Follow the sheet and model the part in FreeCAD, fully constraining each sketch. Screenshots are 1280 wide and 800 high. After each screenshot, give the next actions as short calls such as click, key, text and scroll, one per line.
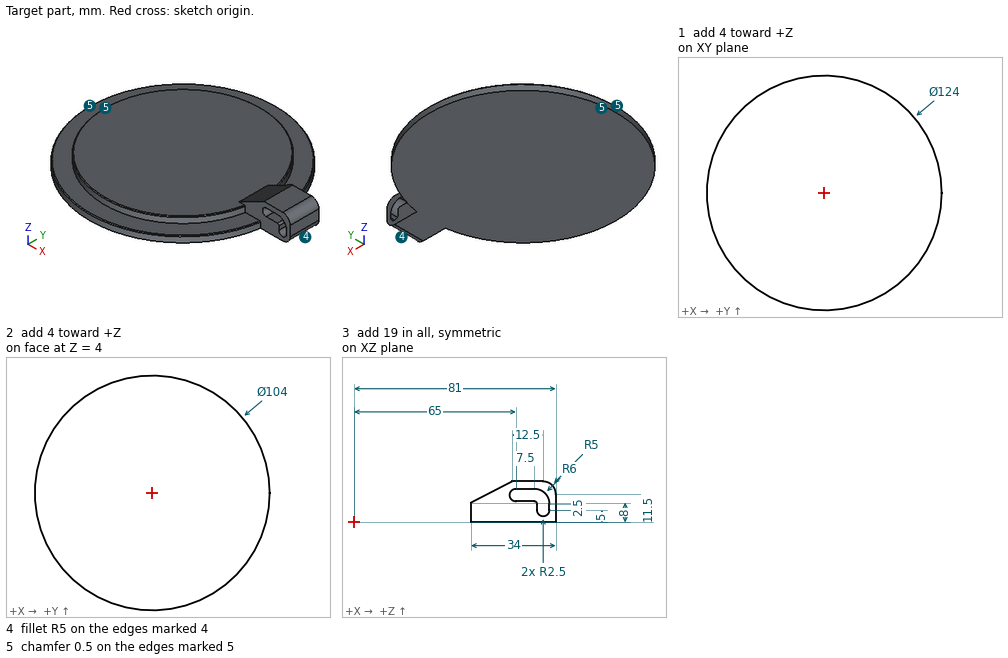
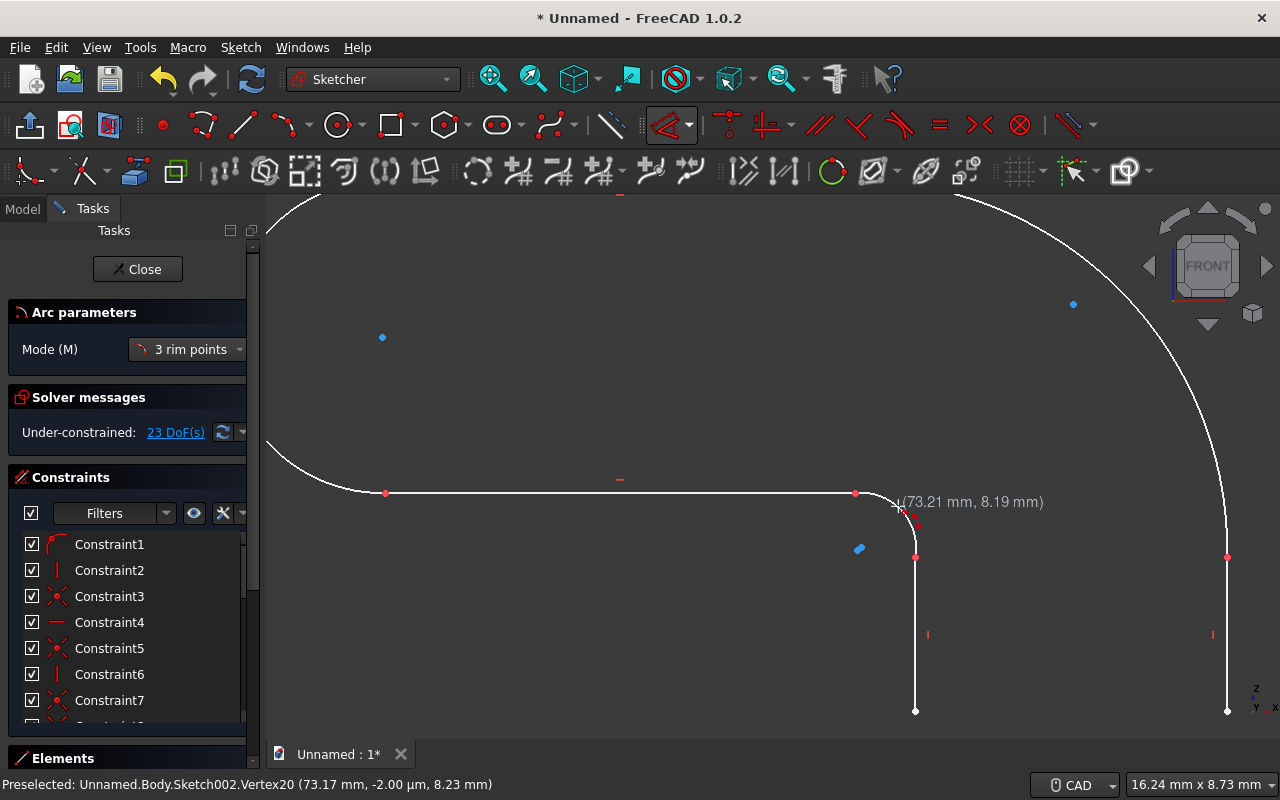
scroll(935, 462, down, 11)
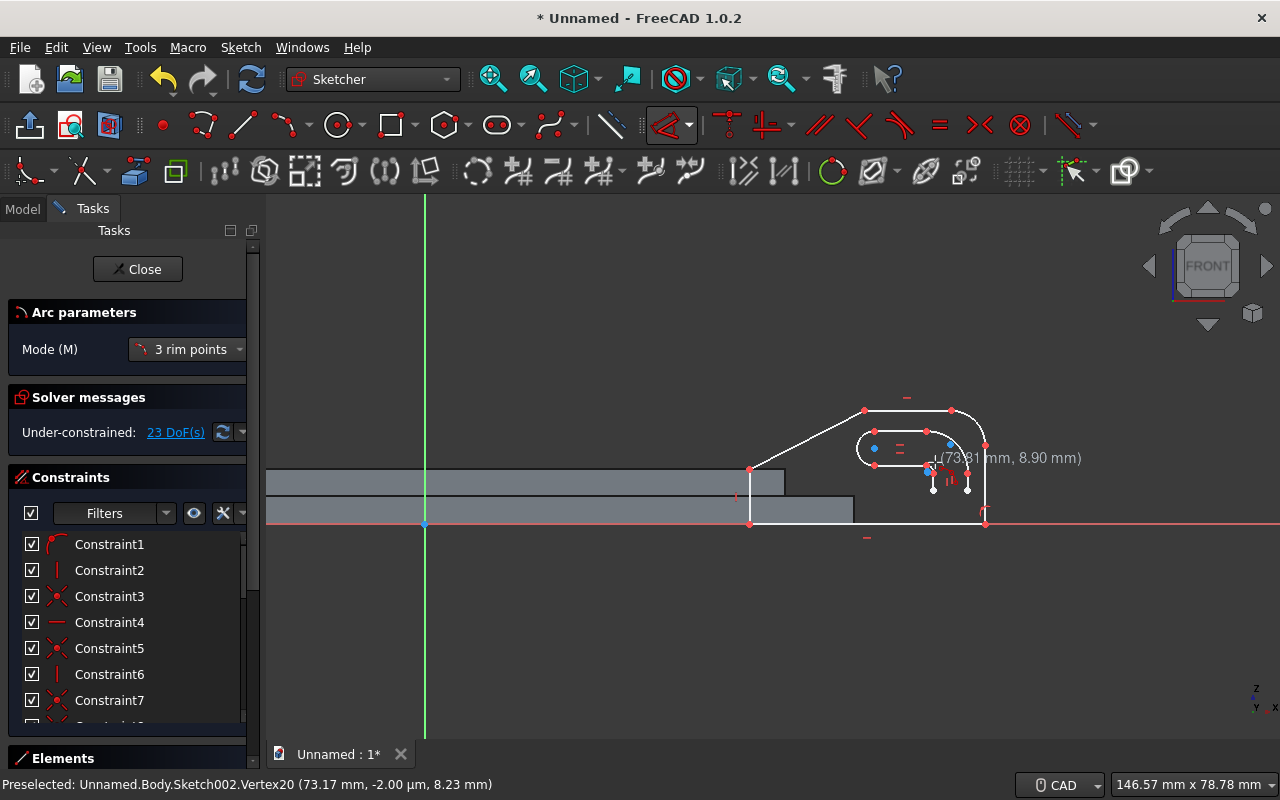
scroll(933, 490, up, 4)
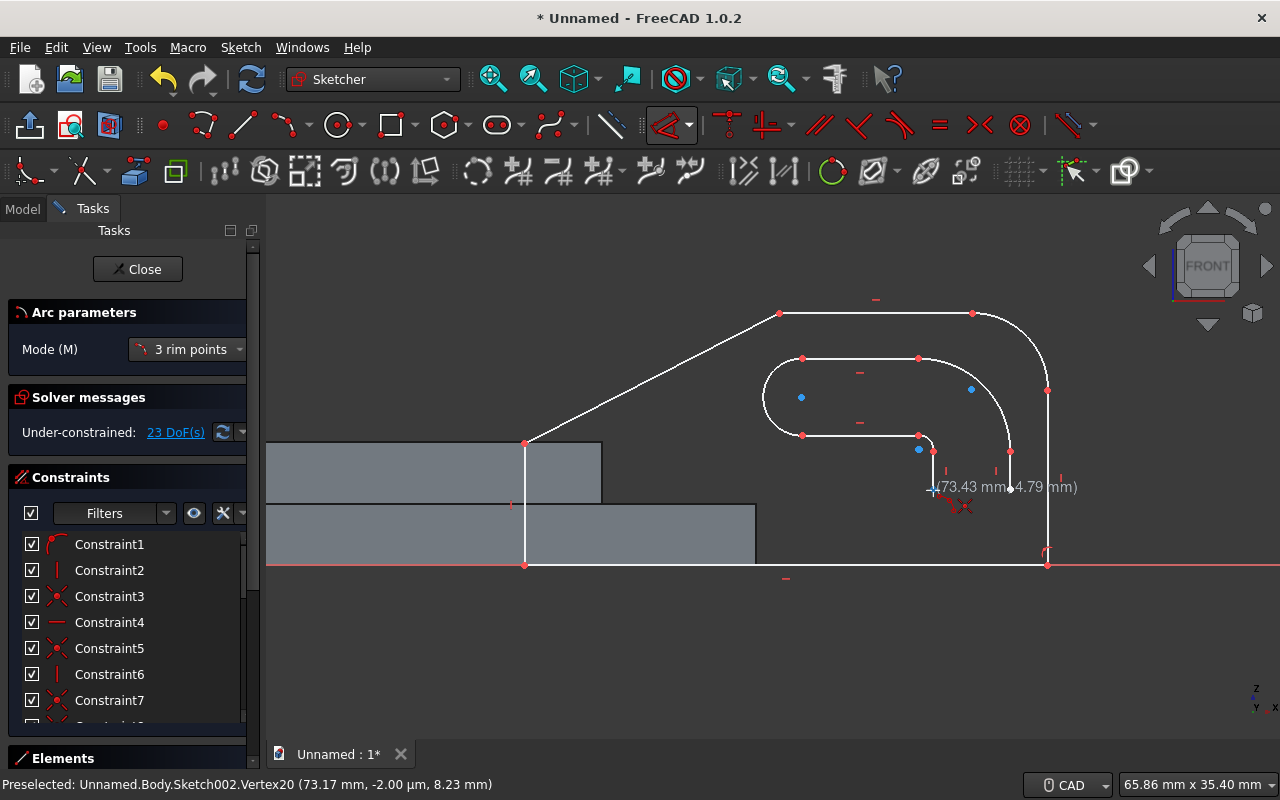
click(933, 489)
click(1010, 489)
click(972, 527)
key(Escape)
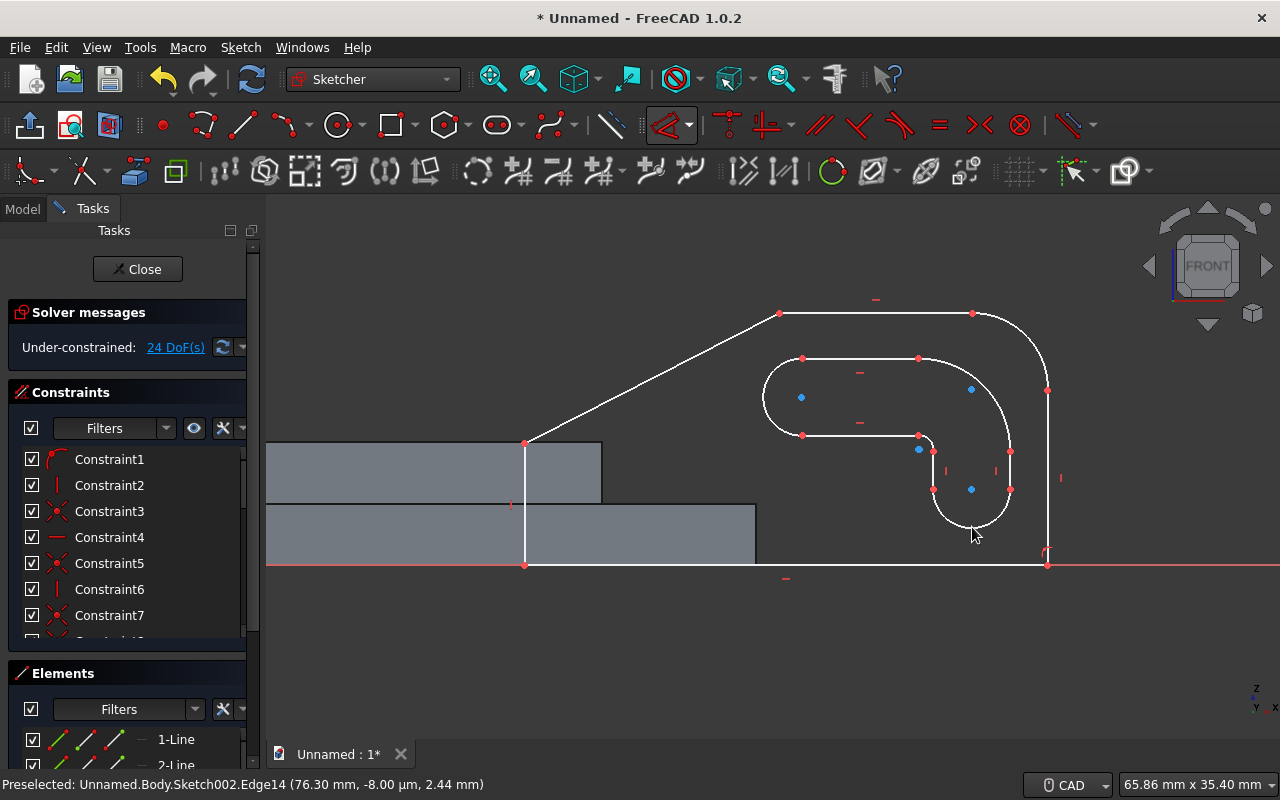
click(1048, 443)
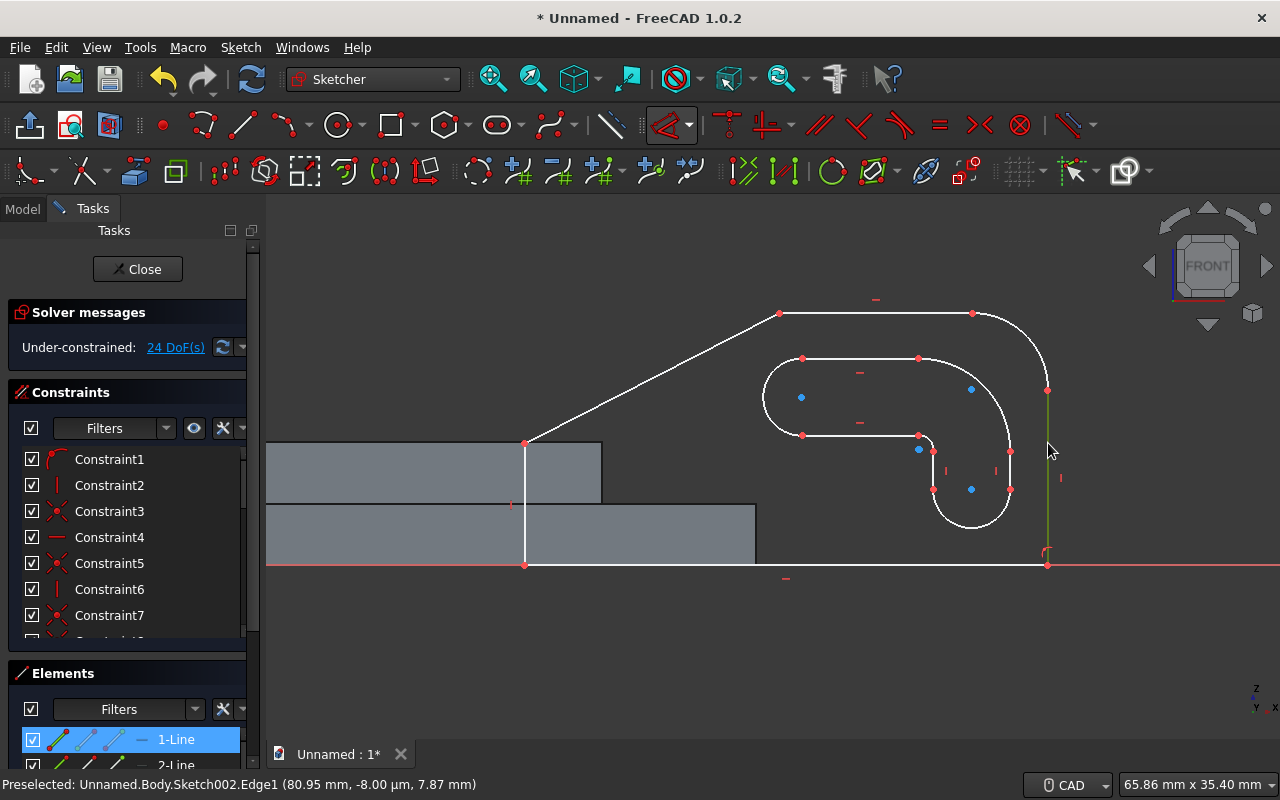
click(1040, 356)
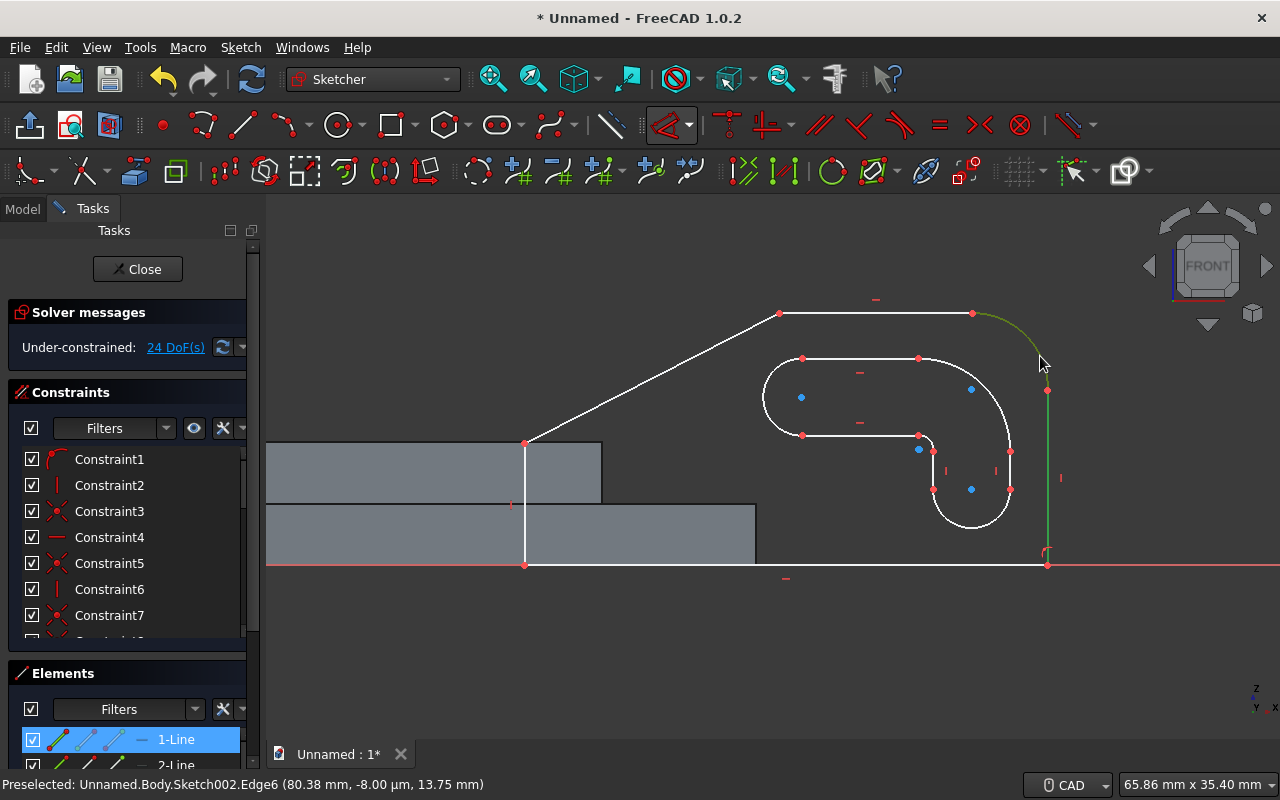
click(900, 126)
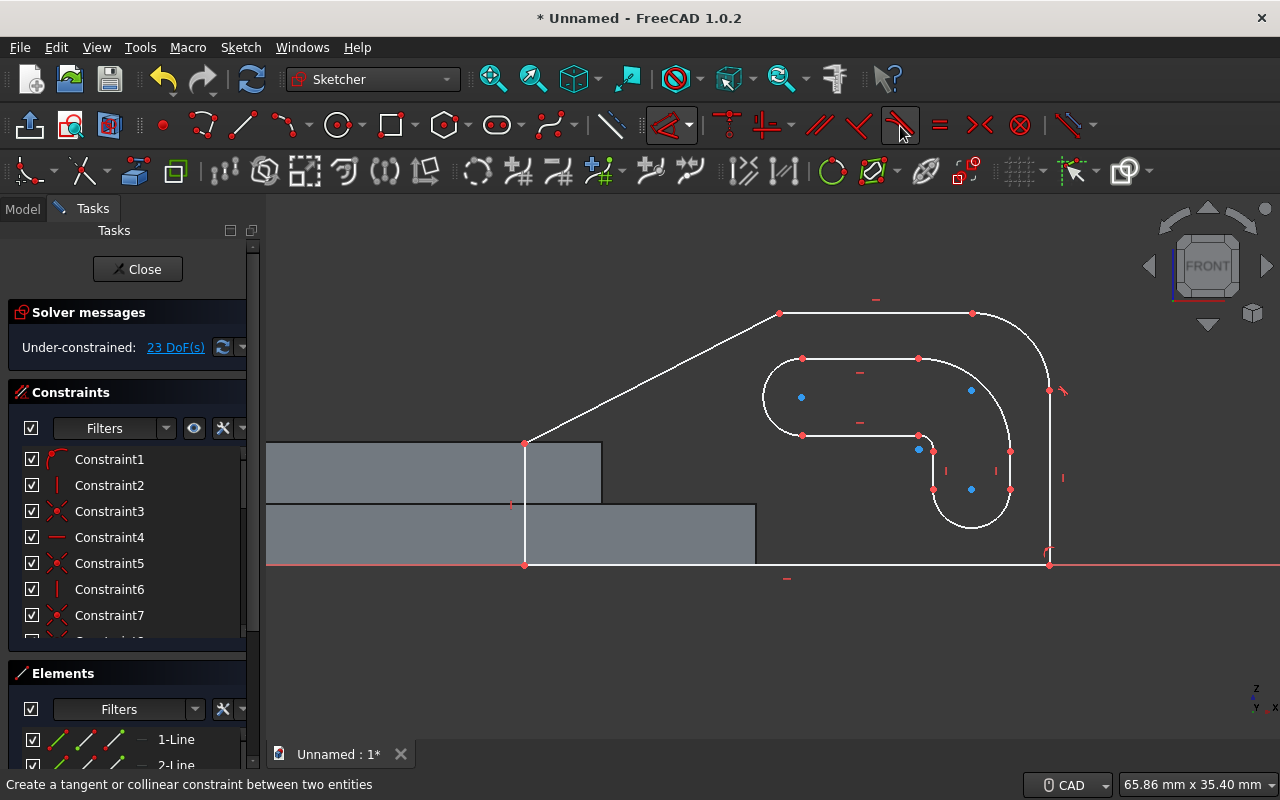
click(838, 313)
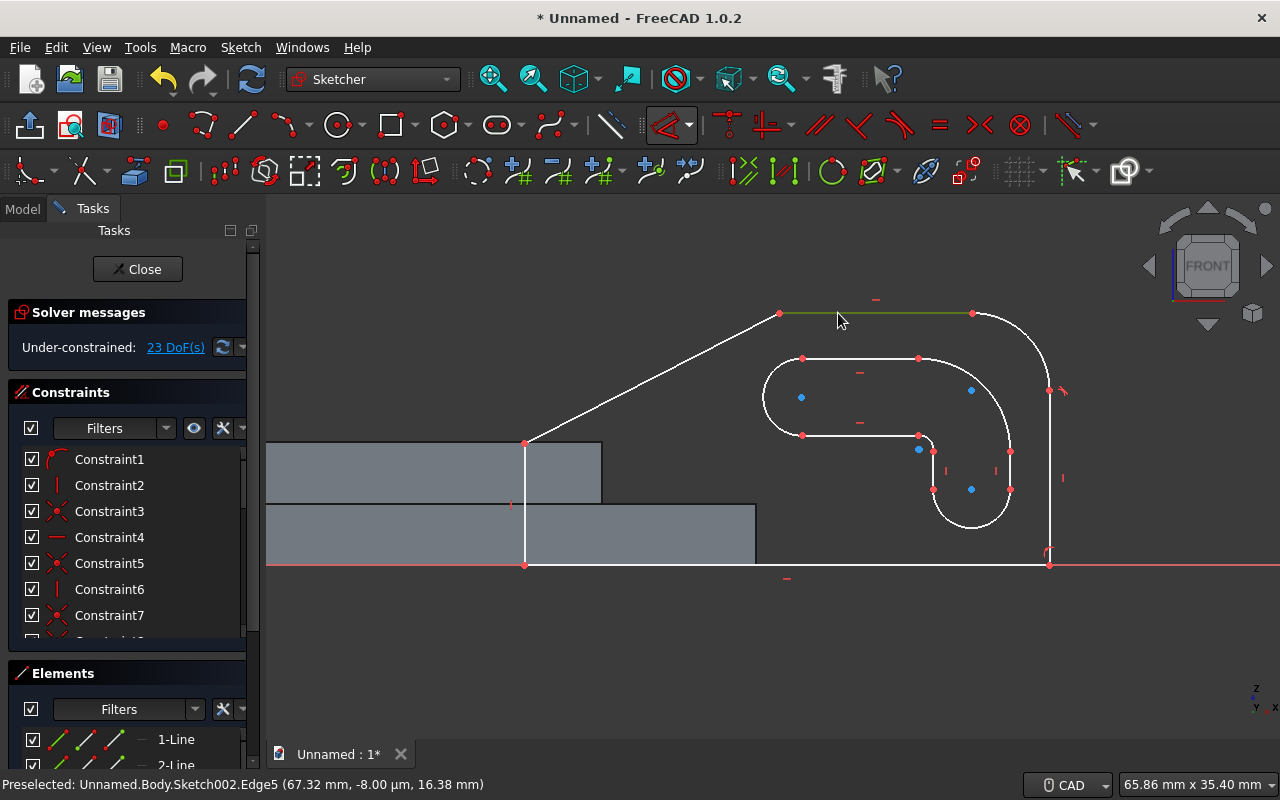
click(1041, 356)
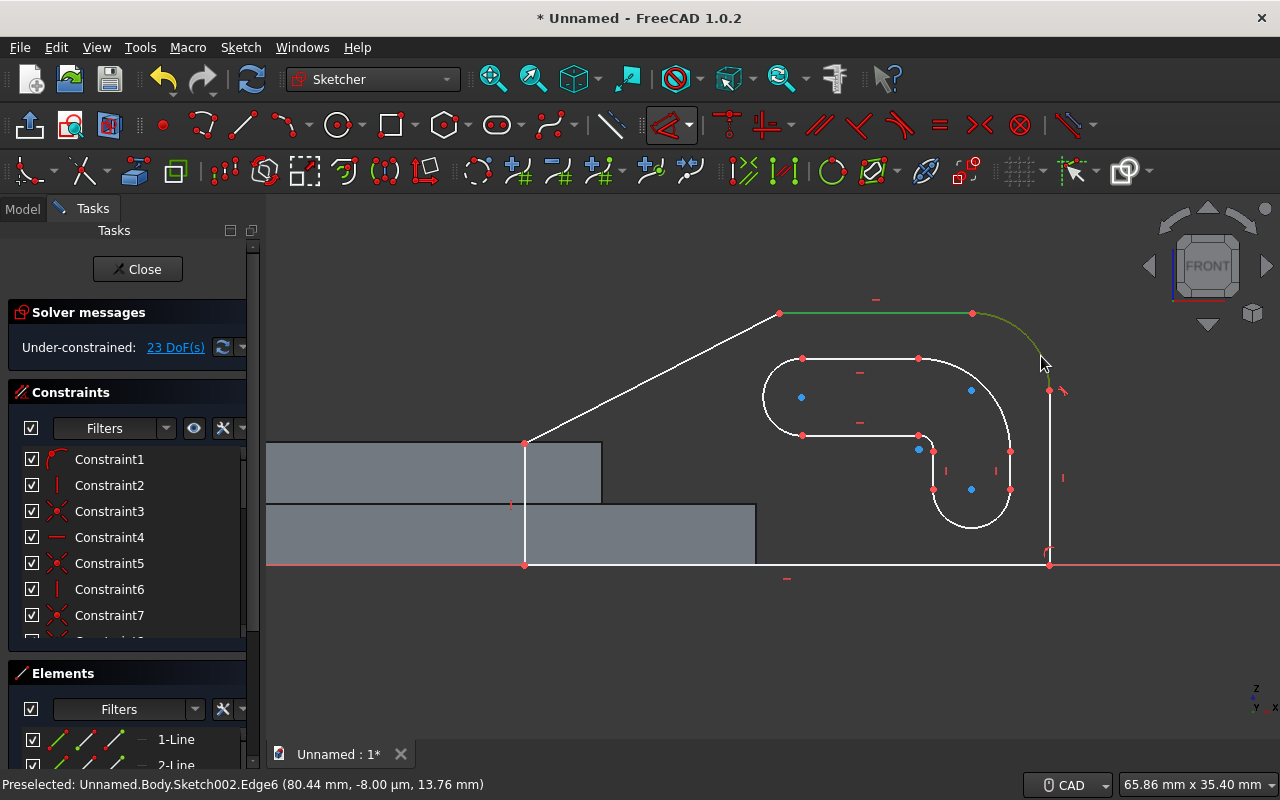
key(t)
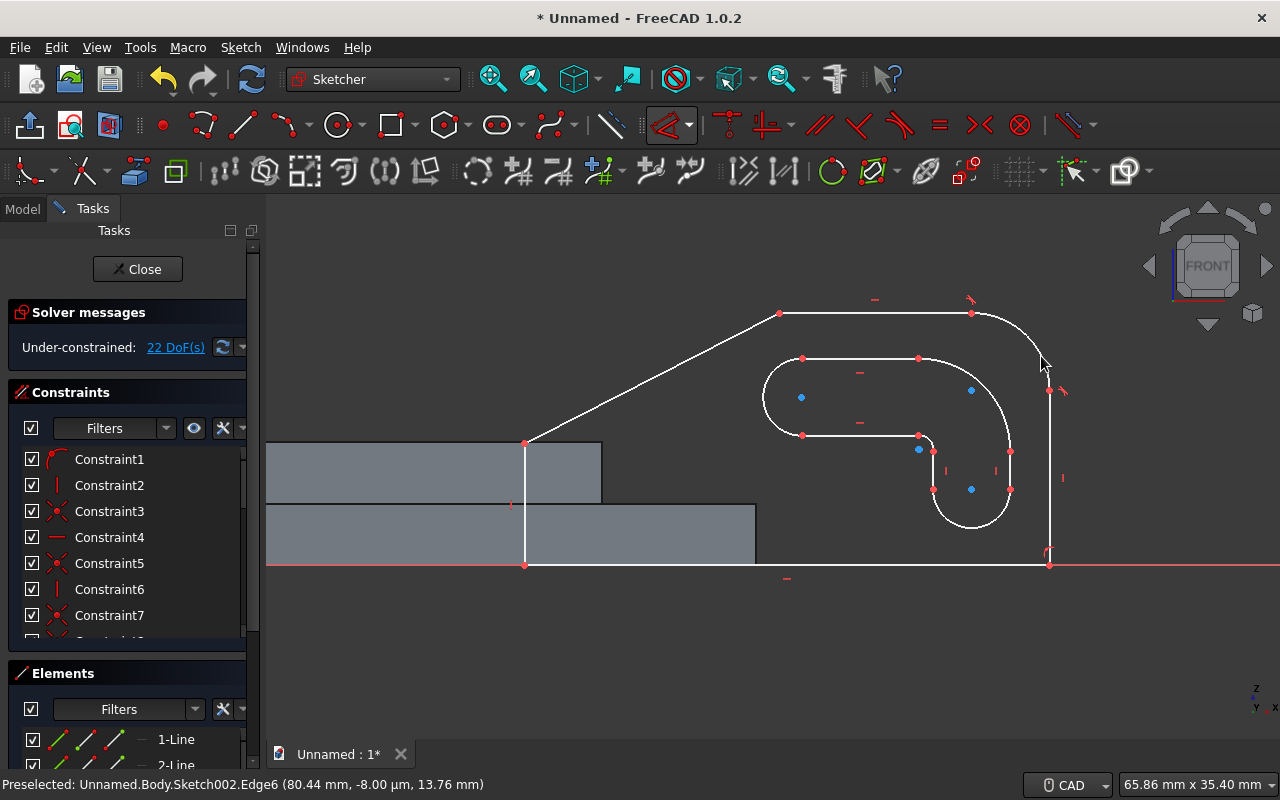
click(1010, 478)